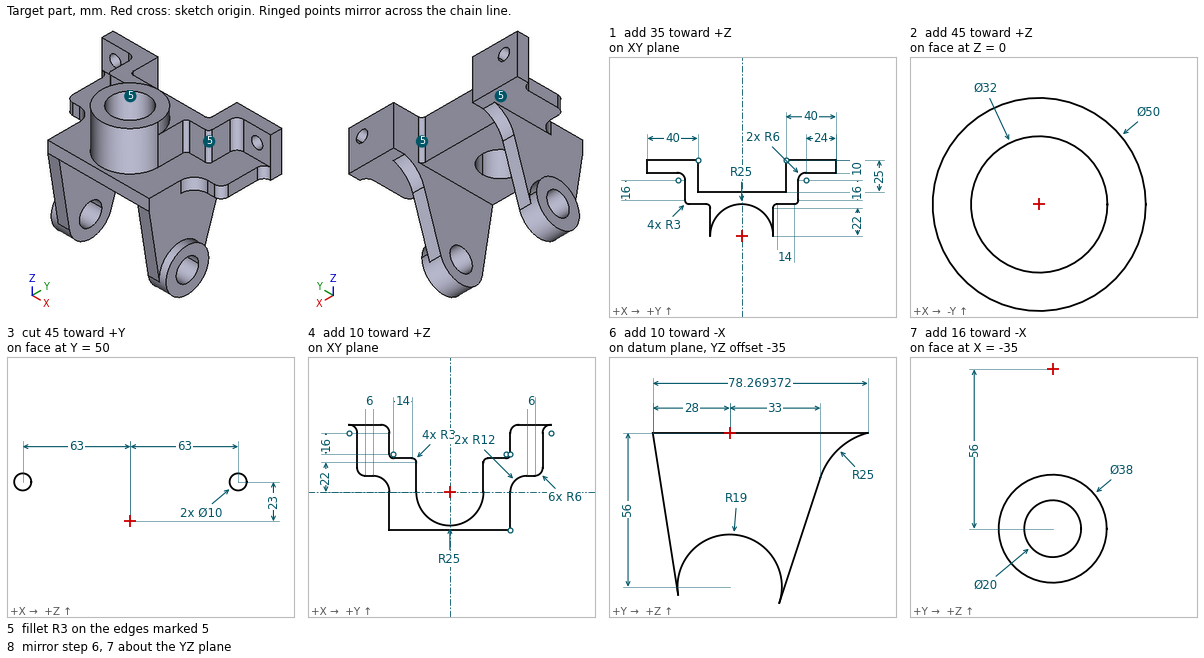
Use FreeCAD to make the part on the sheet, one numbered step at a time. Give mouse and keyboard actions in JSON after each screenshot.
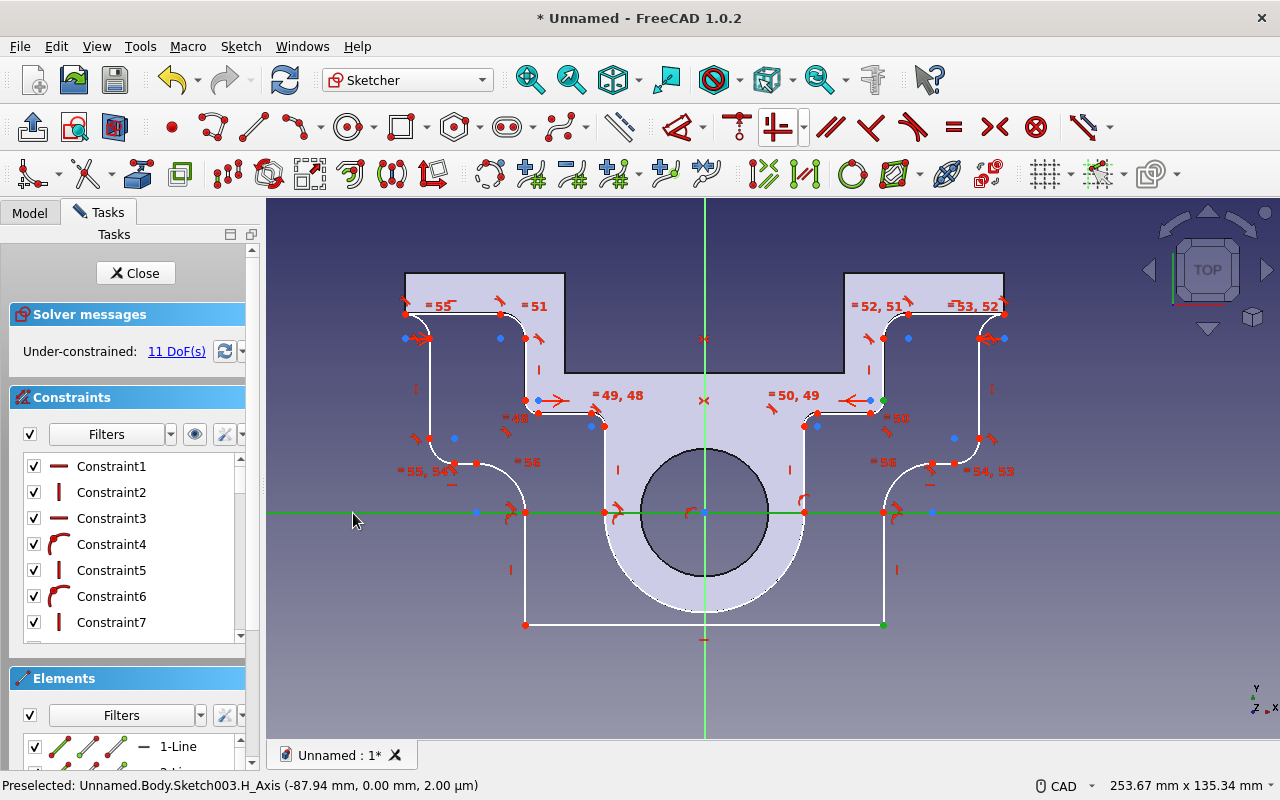
{"action": "left_click", "coordinate": [995, 128]}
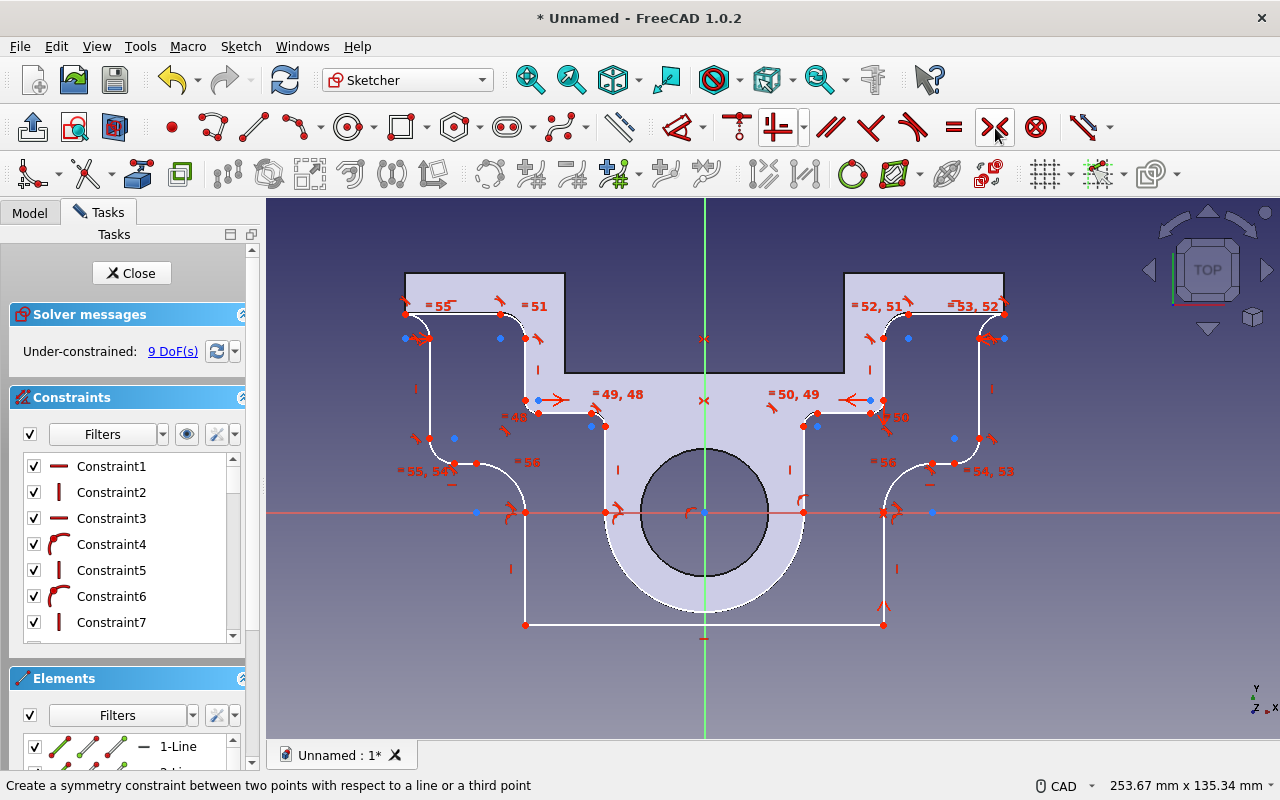
{"action": "left_click", "coordinate": [676, 128]}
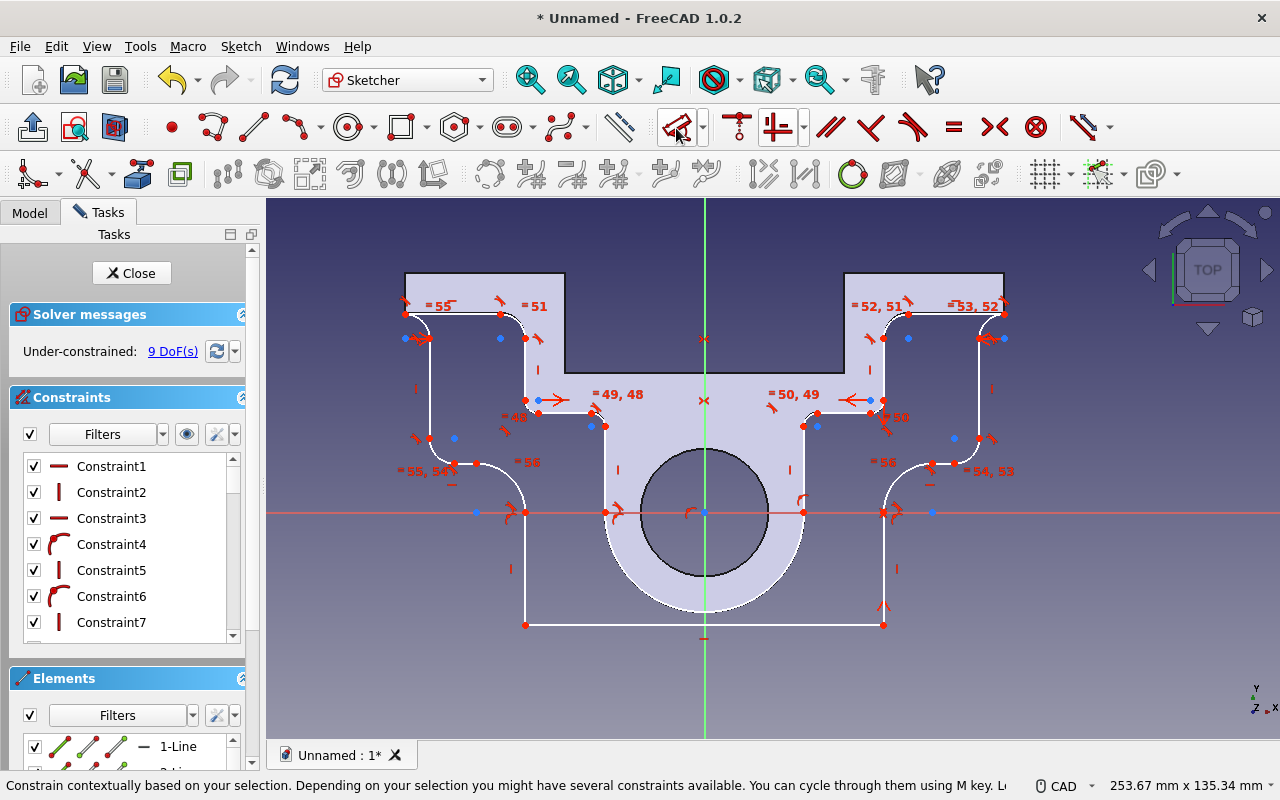
{"action": "scroll", "coordinate": [523, 328], "scroll_direction": "up", "scroll_amount": 3}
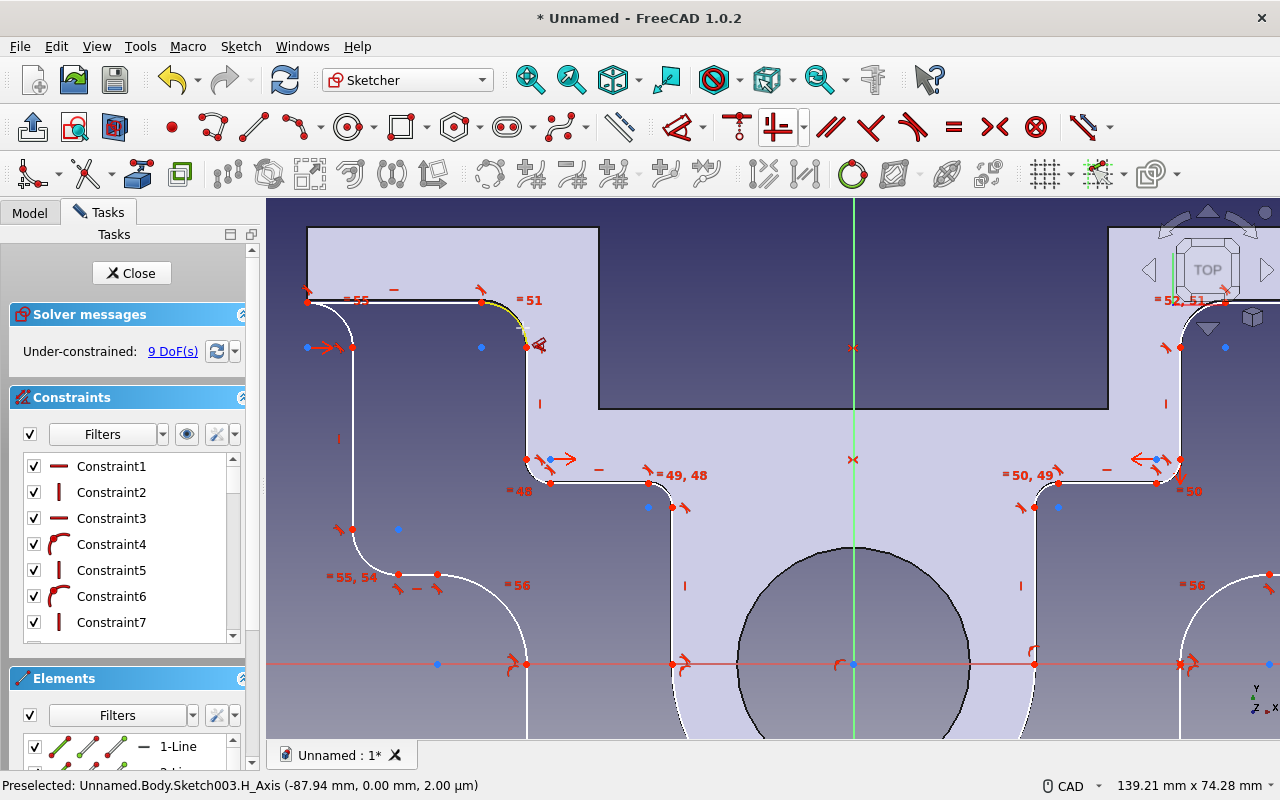
{"action": "left_click", "coordinate": [522, 327]}
{"action": "left_click", "coordinate": [550, 312]}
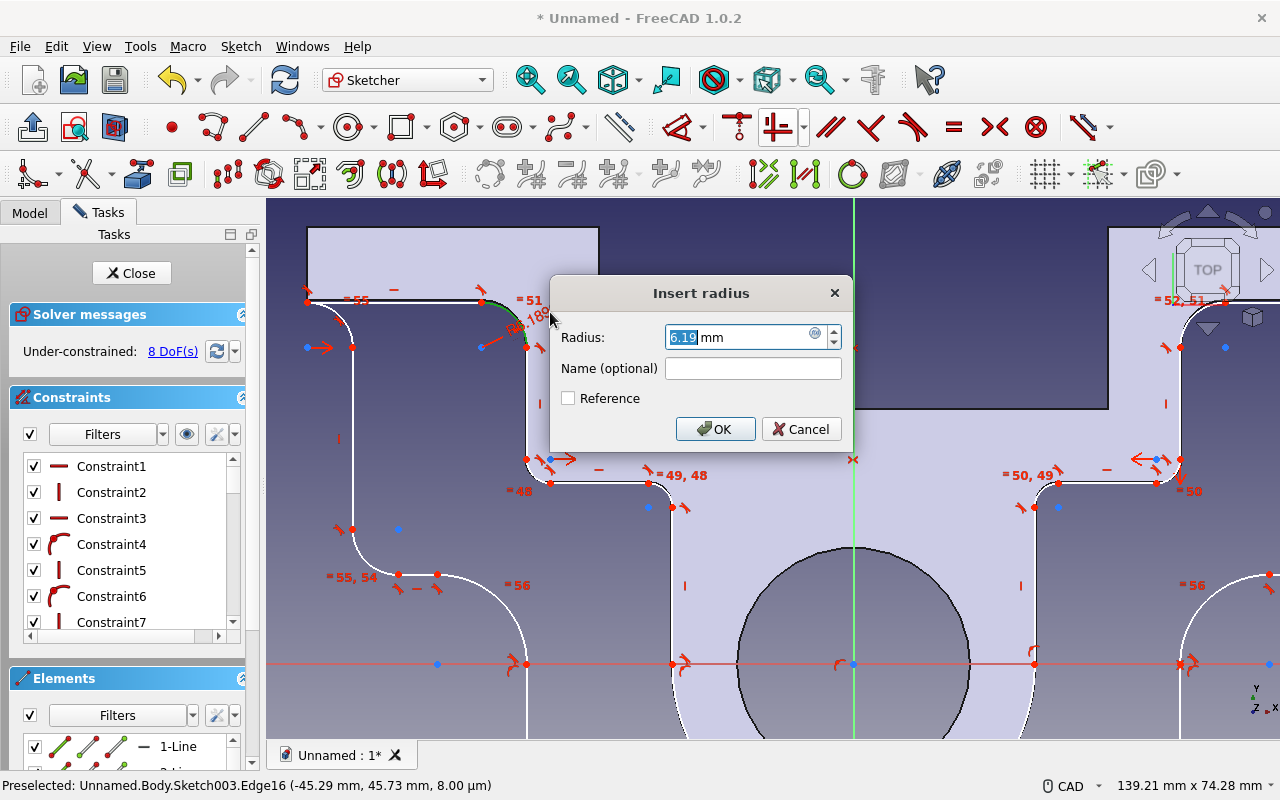
{"action": "type", "text": "6"}
{"action": "key", "text": "Return"}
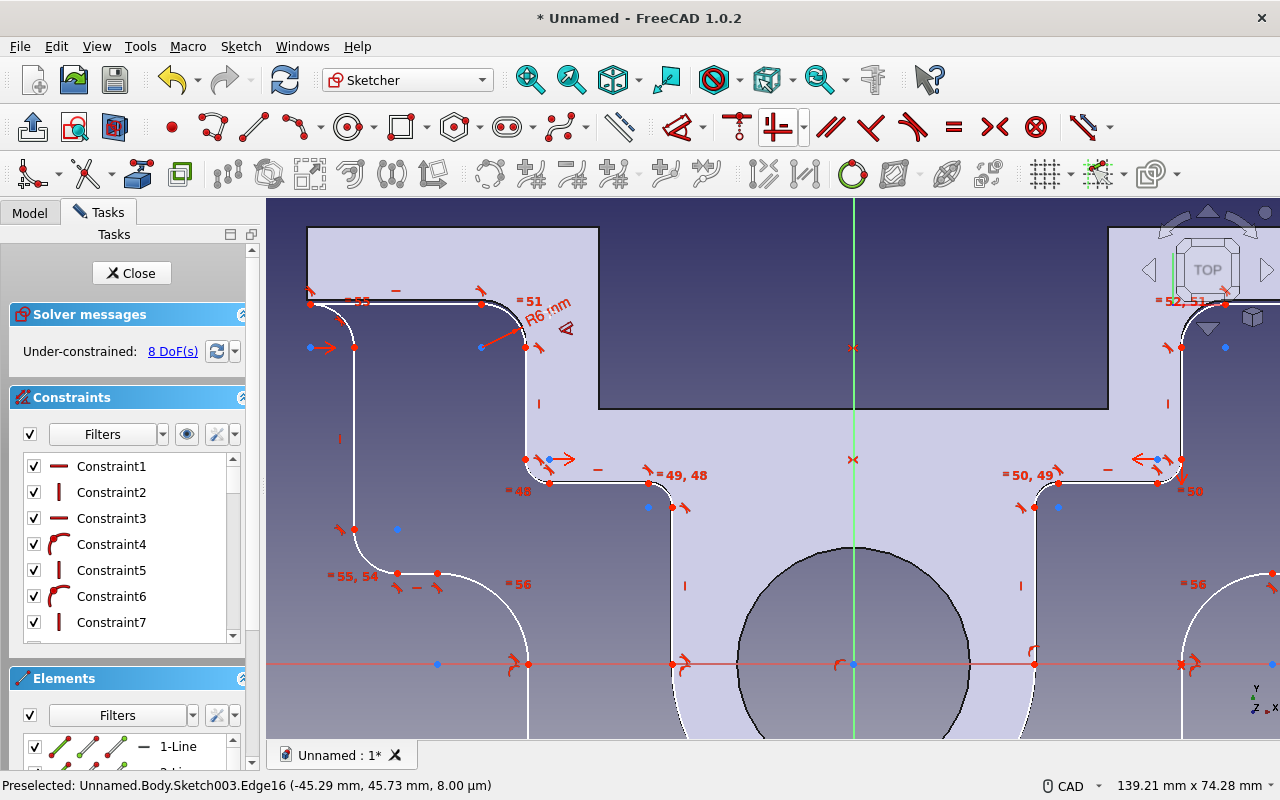
{"action": "scroll", "coordinate": [528, 470], "scroll_direction": "up", "scroll_amount": 3}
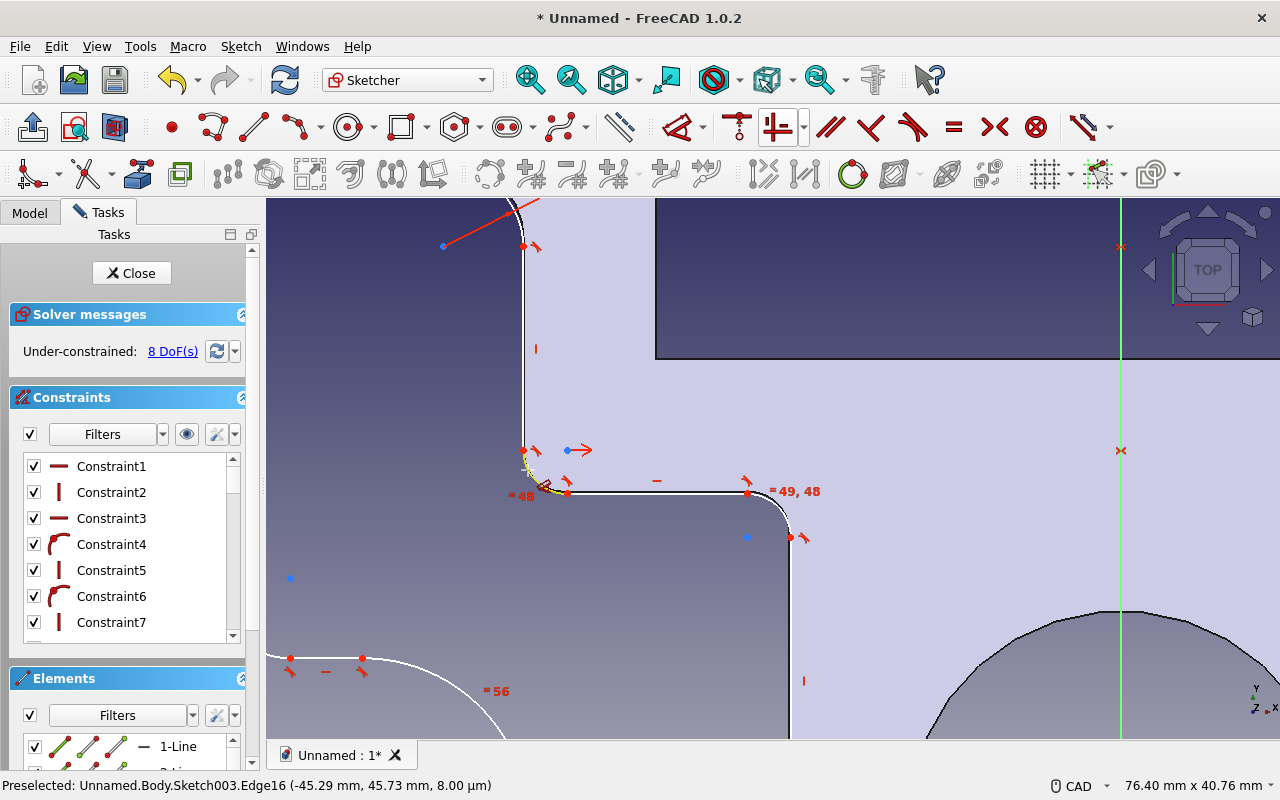
{"action": "left_click", "coordinate": [528, 470]}
{"action": "left_click", "coordinate": [499, 485]}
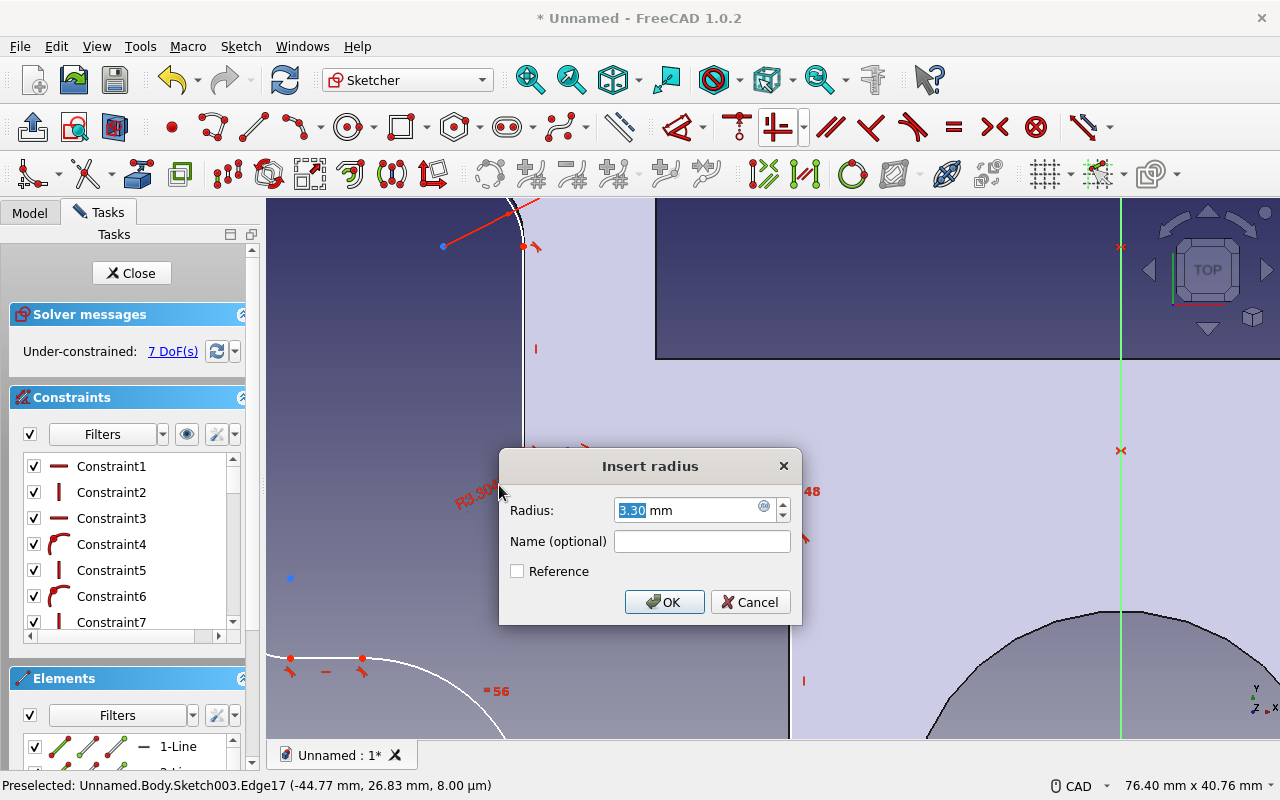
{"action": "type", "text": "3"}
{"action": "key", "text": "Return"}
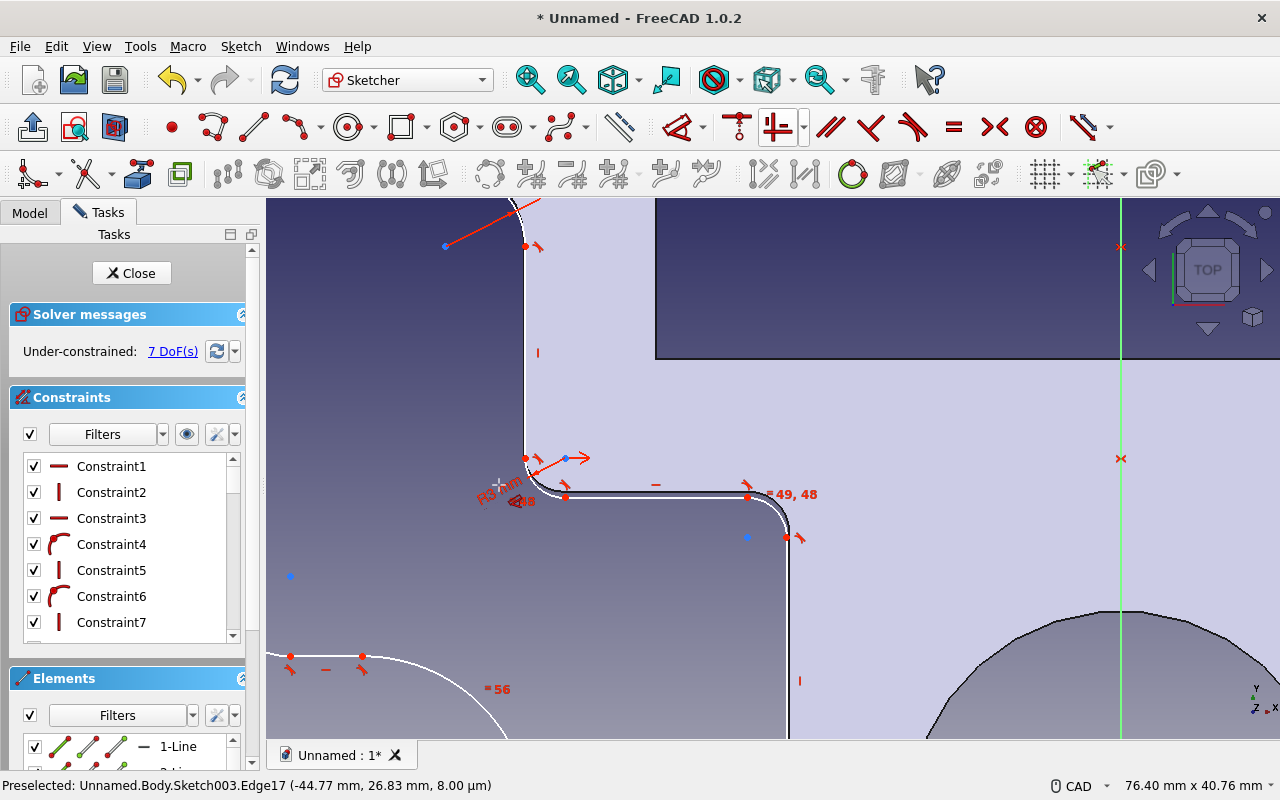
{"action": "scroll", "coordinate": [525, 378], "scroll_direction": "down", "scroll_amount": 6}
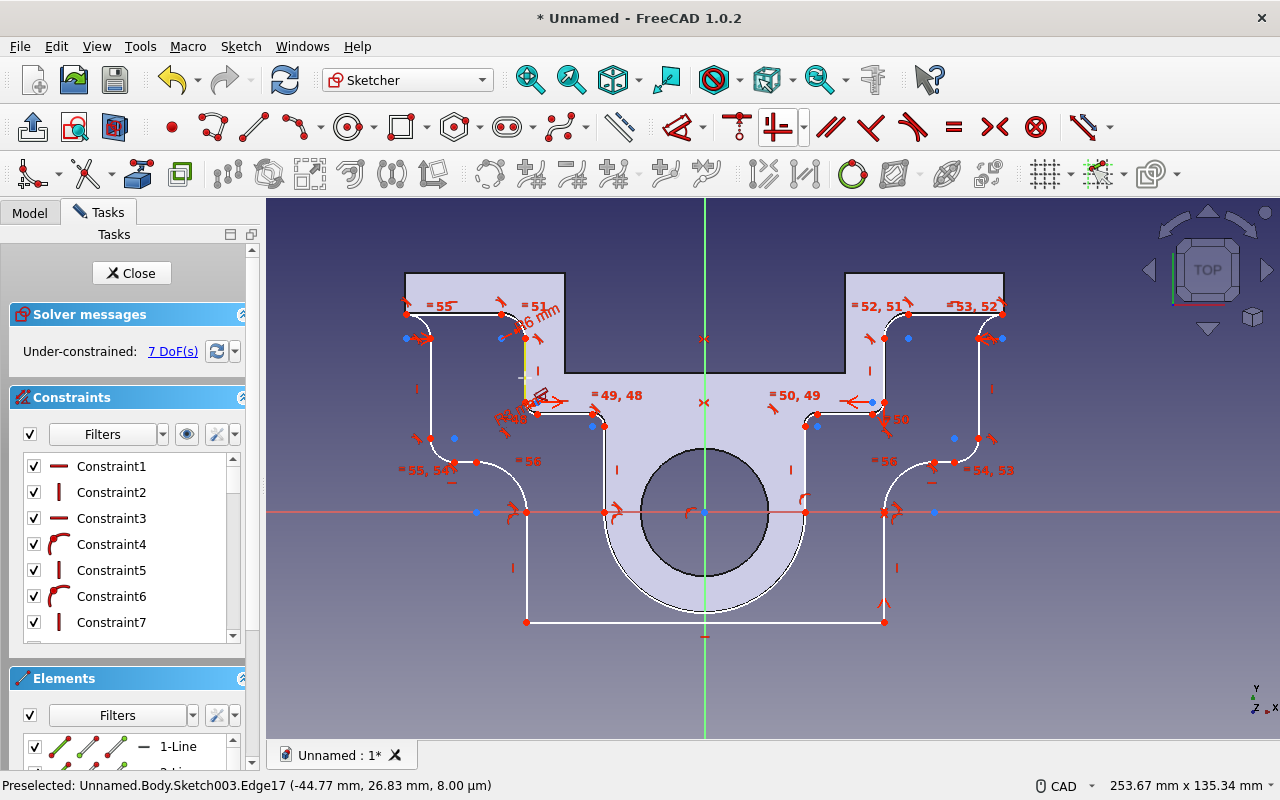
{"action": "left_click", "coordinate": [646, 594]}
{"action": "left_click", "coordinate": [585, 570]}